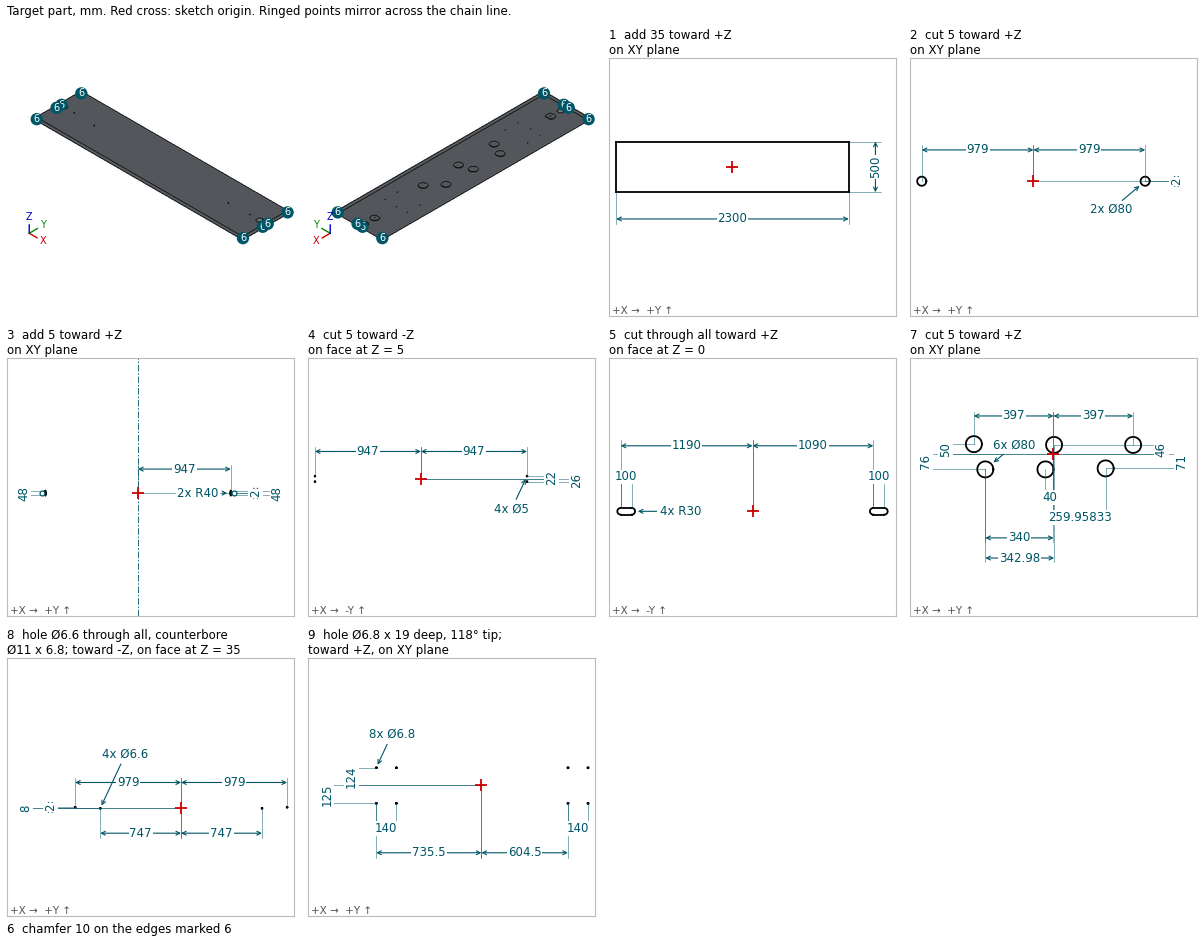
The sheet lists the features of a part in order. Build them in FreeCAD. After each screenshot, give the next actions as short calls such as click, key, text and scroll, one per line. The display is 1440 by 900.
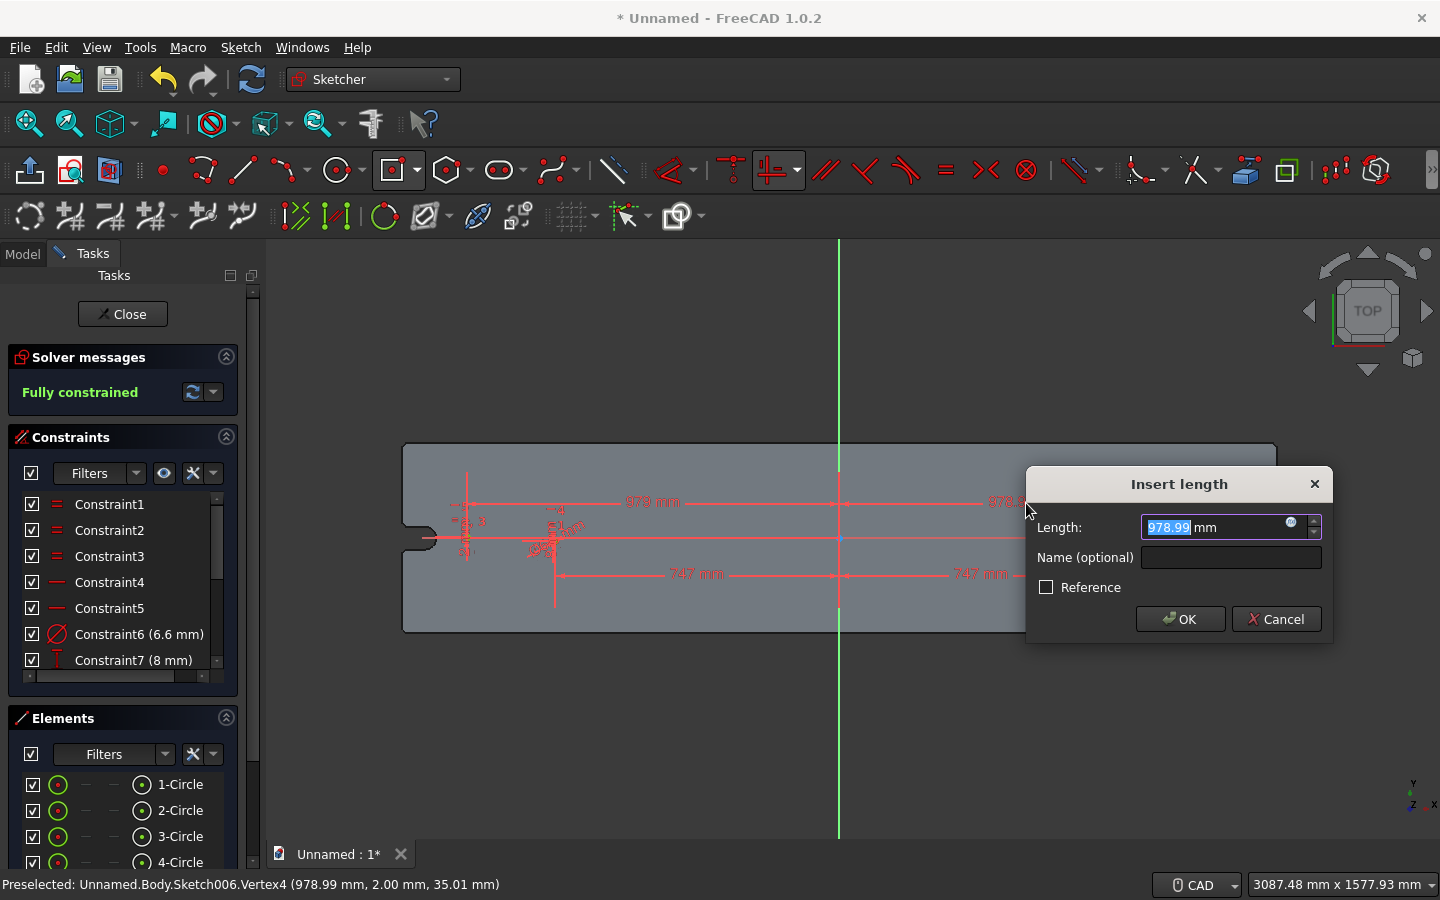
text(979)
key(Return)
key(Escape)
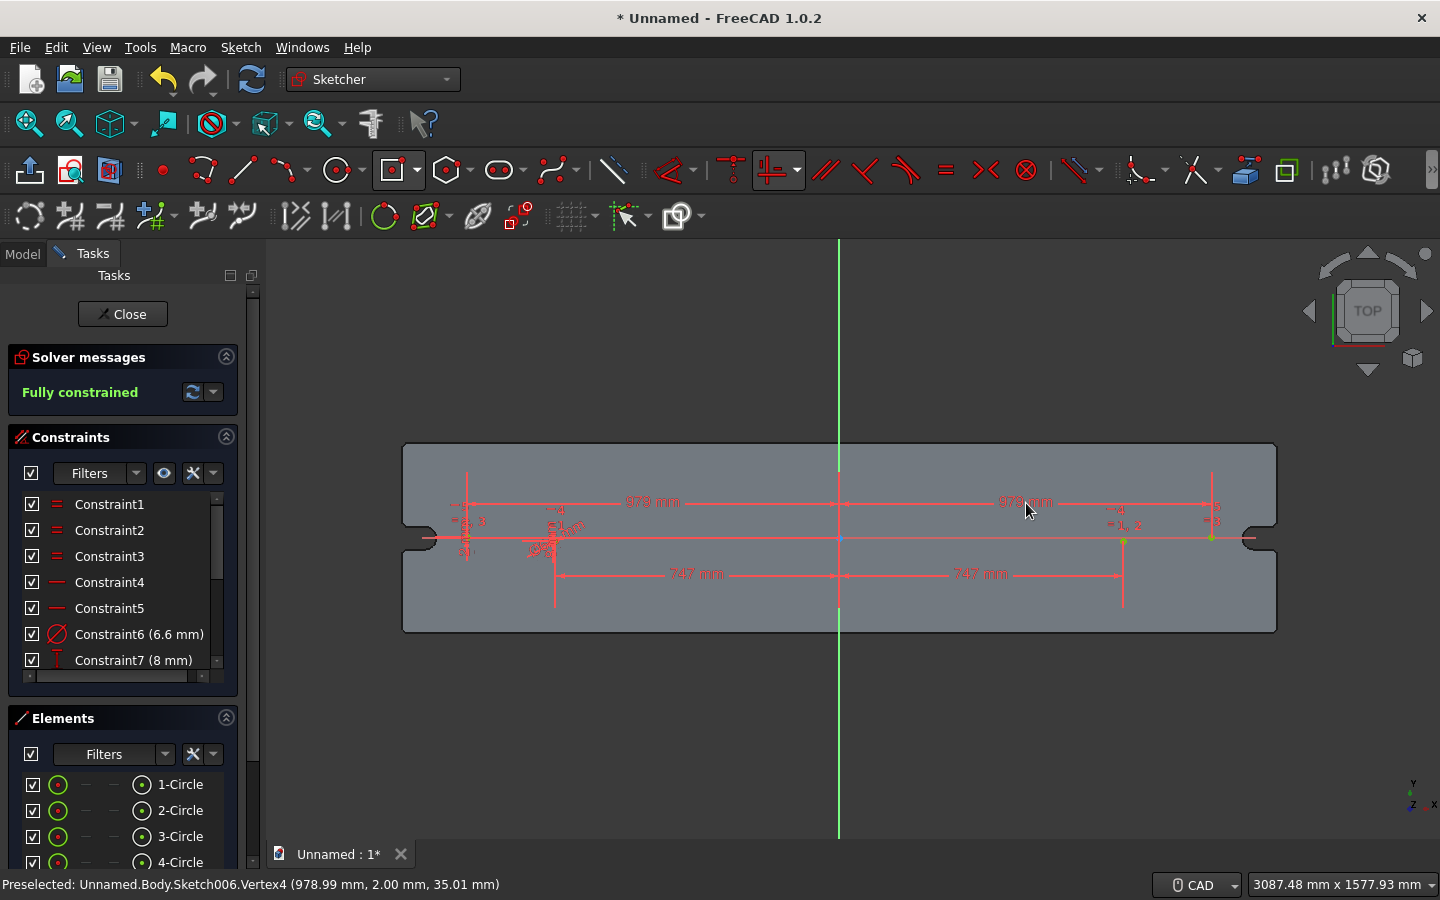
click(123, 314)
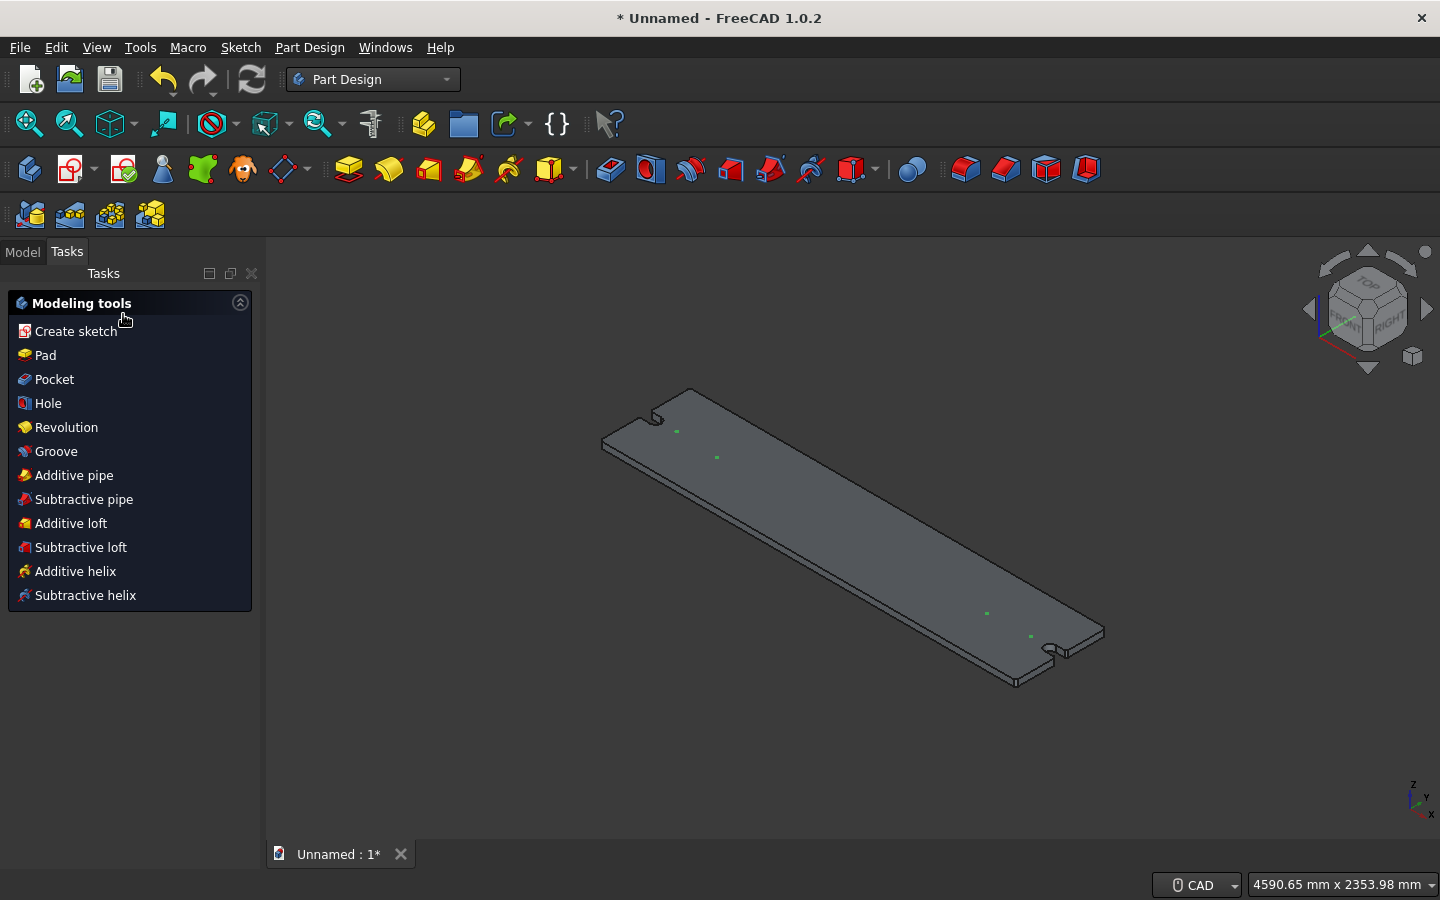
click(652, 170)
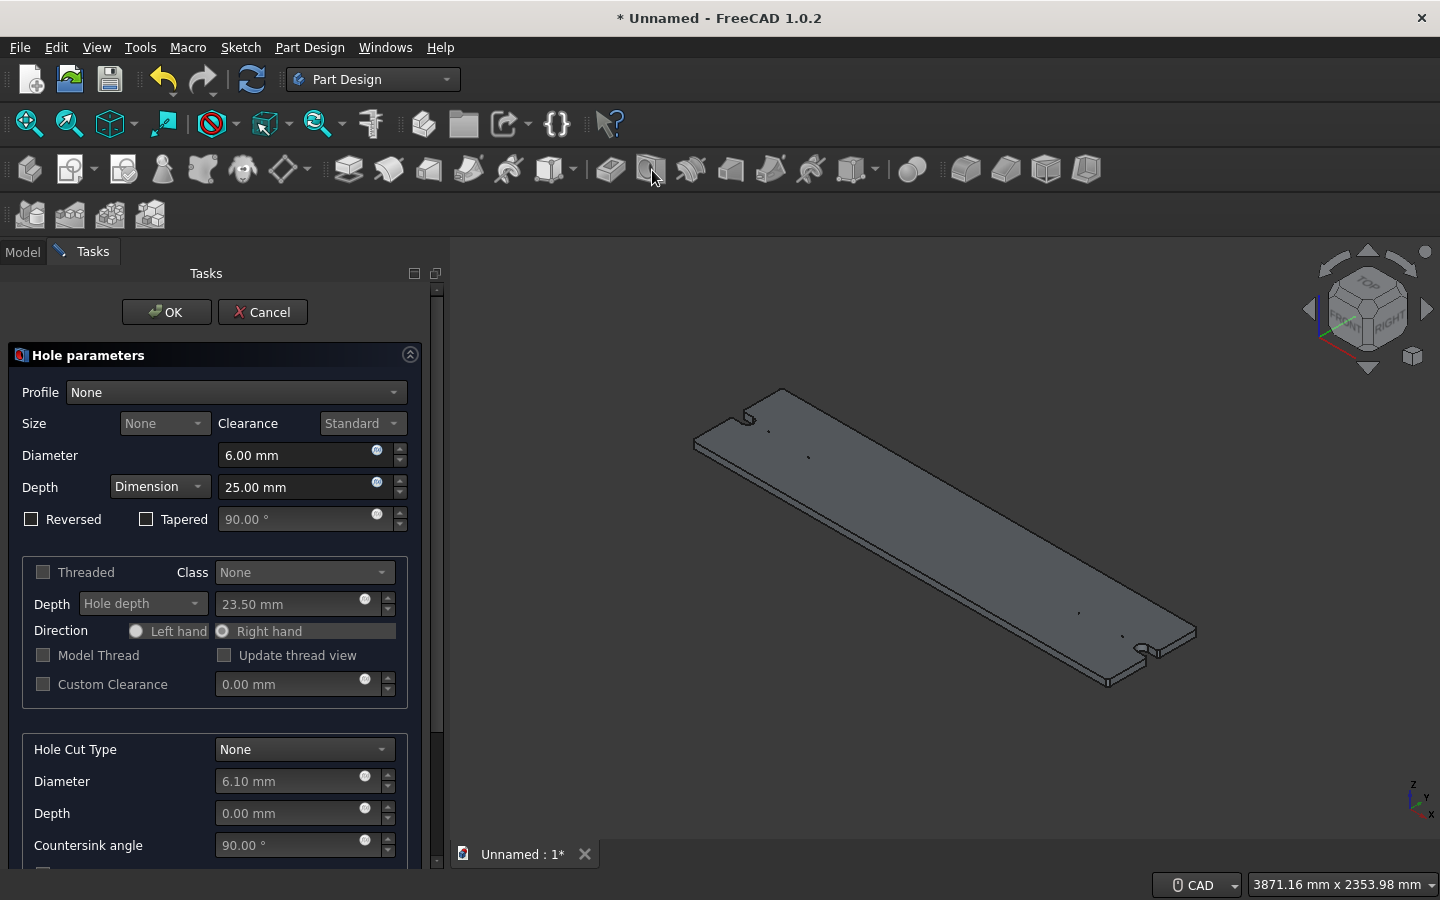
triple_click(305, 455)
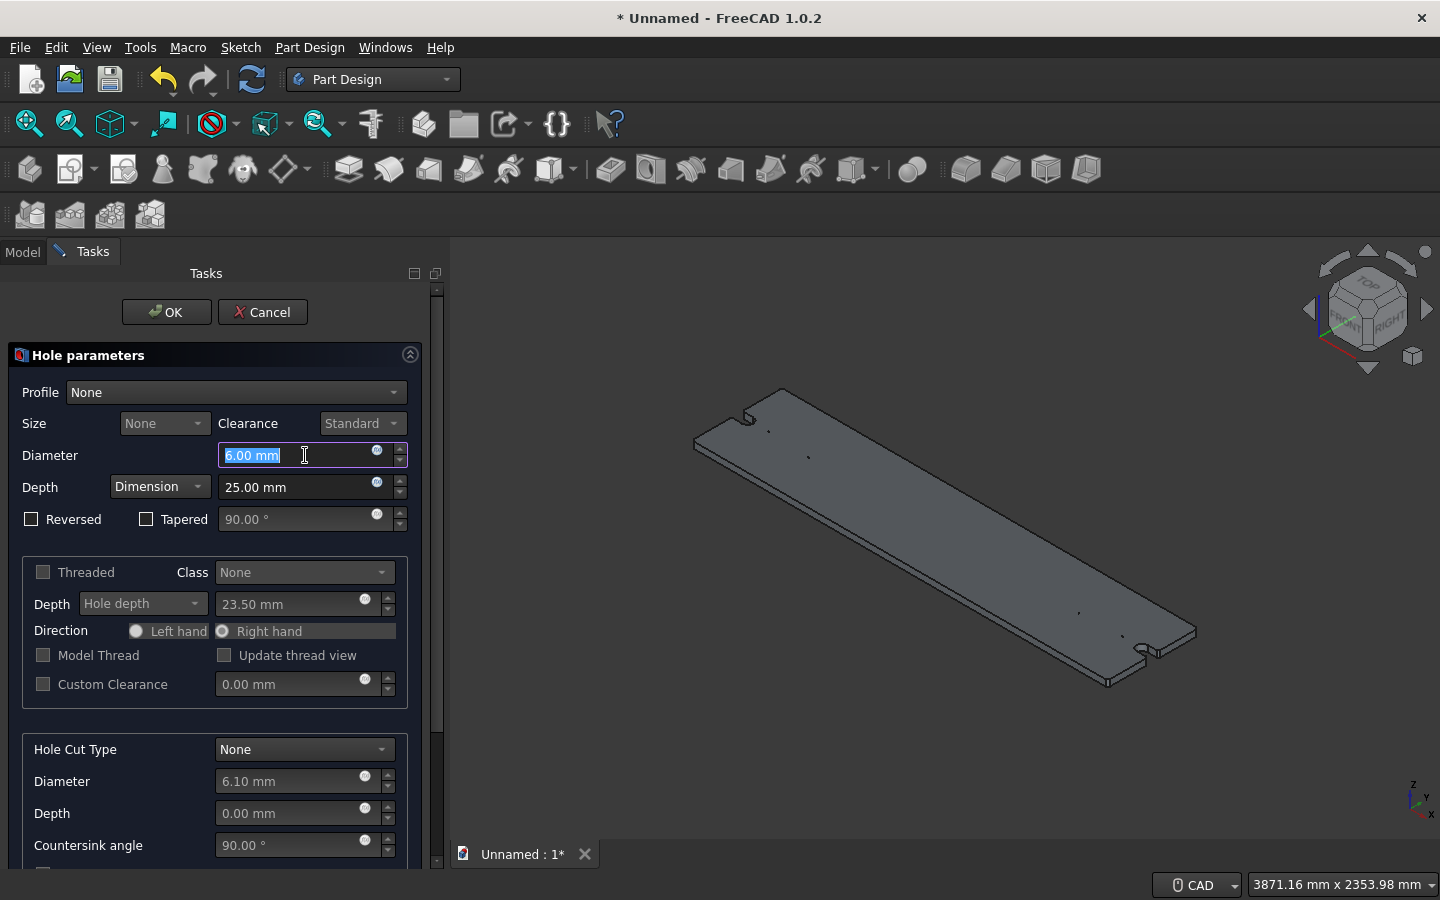
text(6.6)
key(Tab)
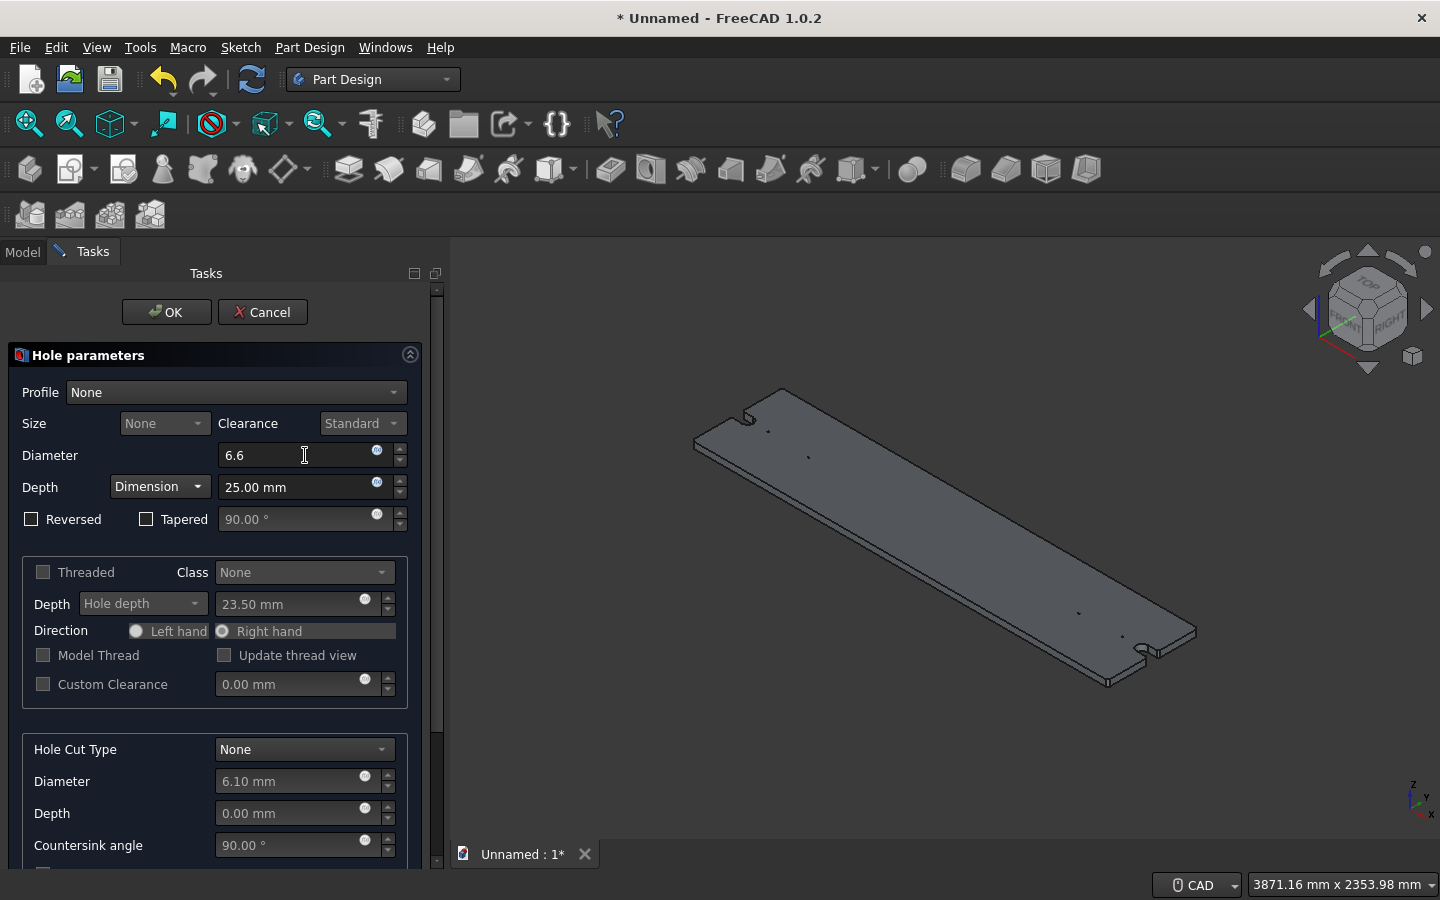
click(161, 486)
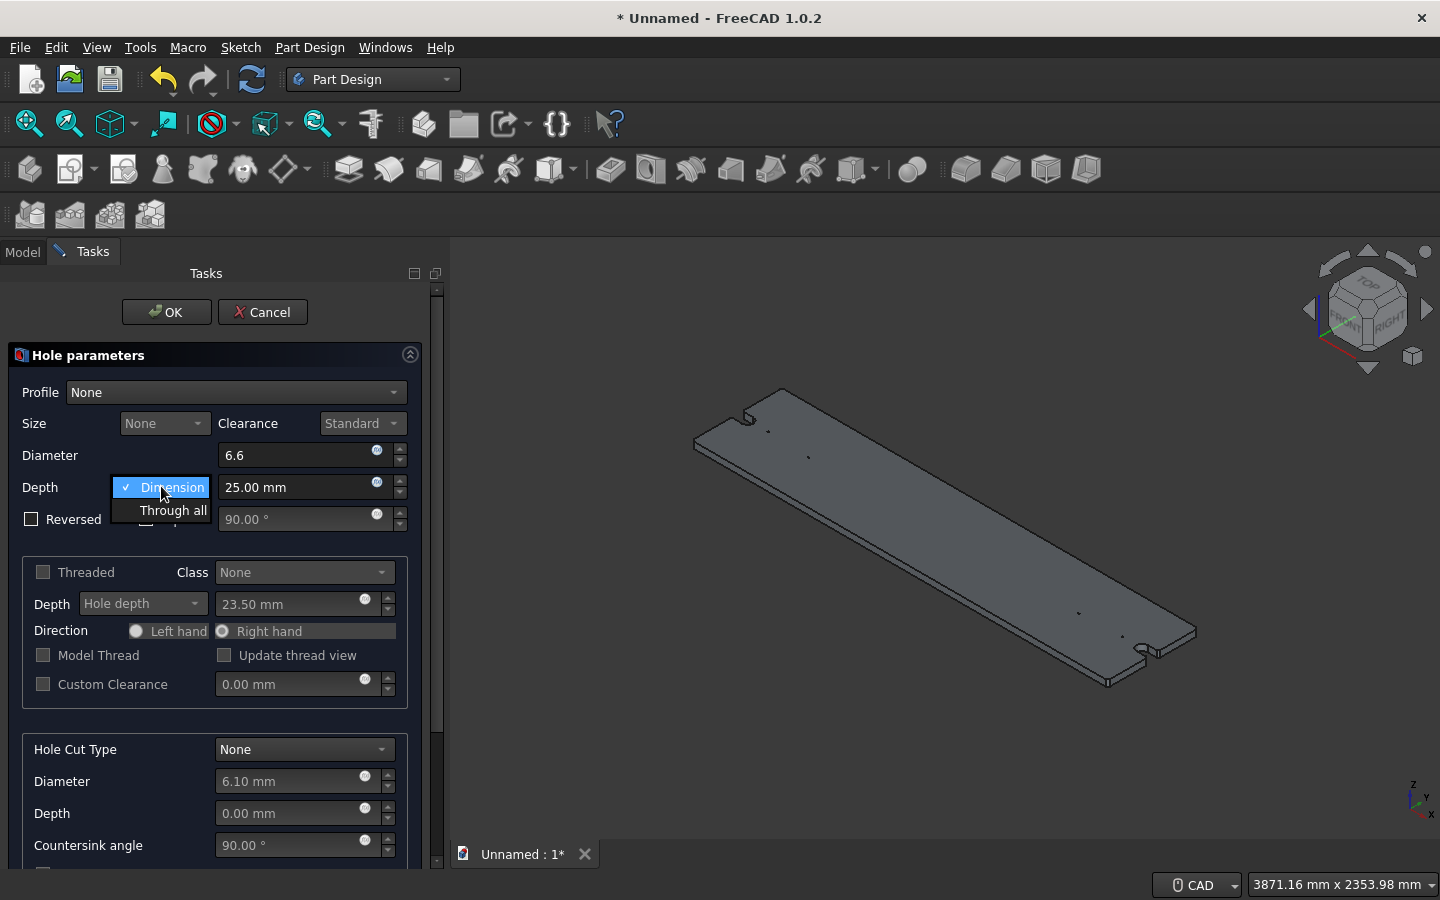
click(160, 510)